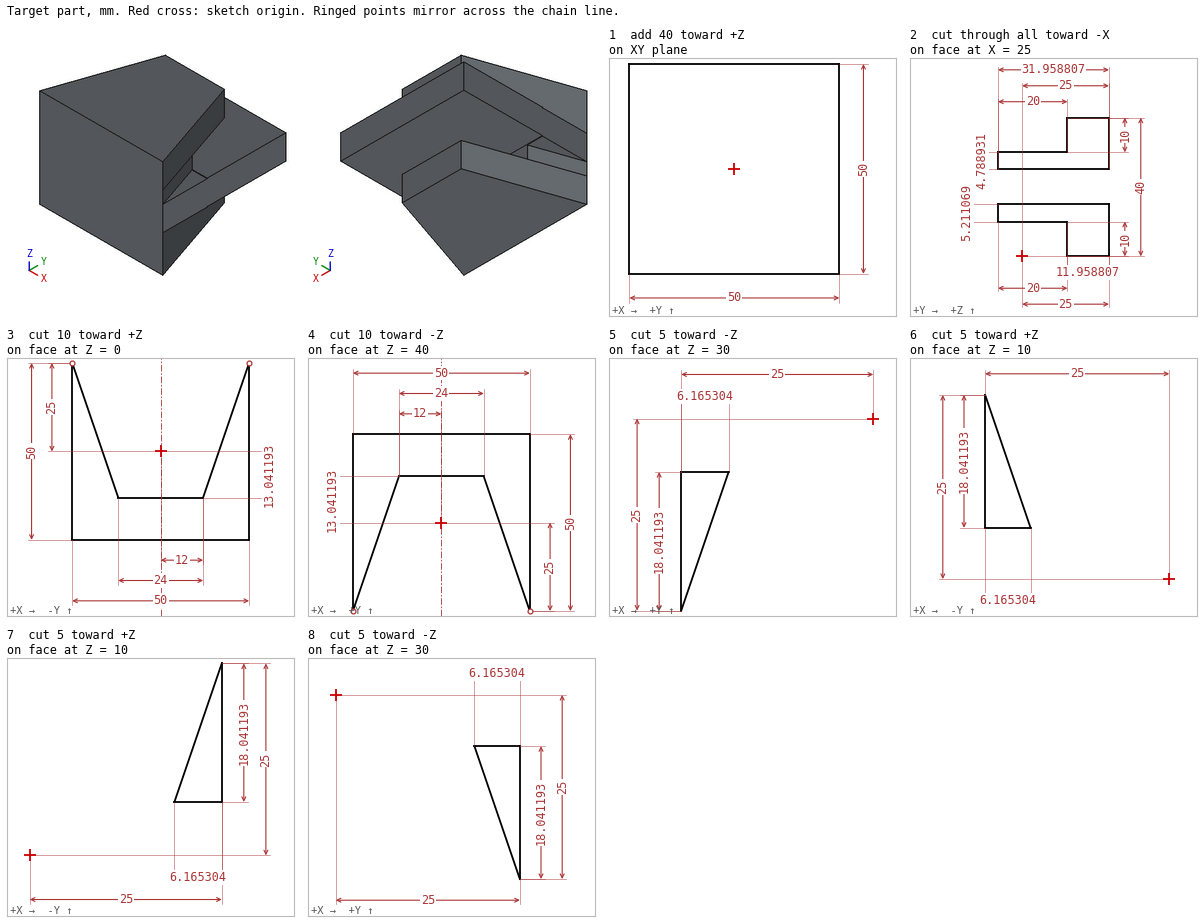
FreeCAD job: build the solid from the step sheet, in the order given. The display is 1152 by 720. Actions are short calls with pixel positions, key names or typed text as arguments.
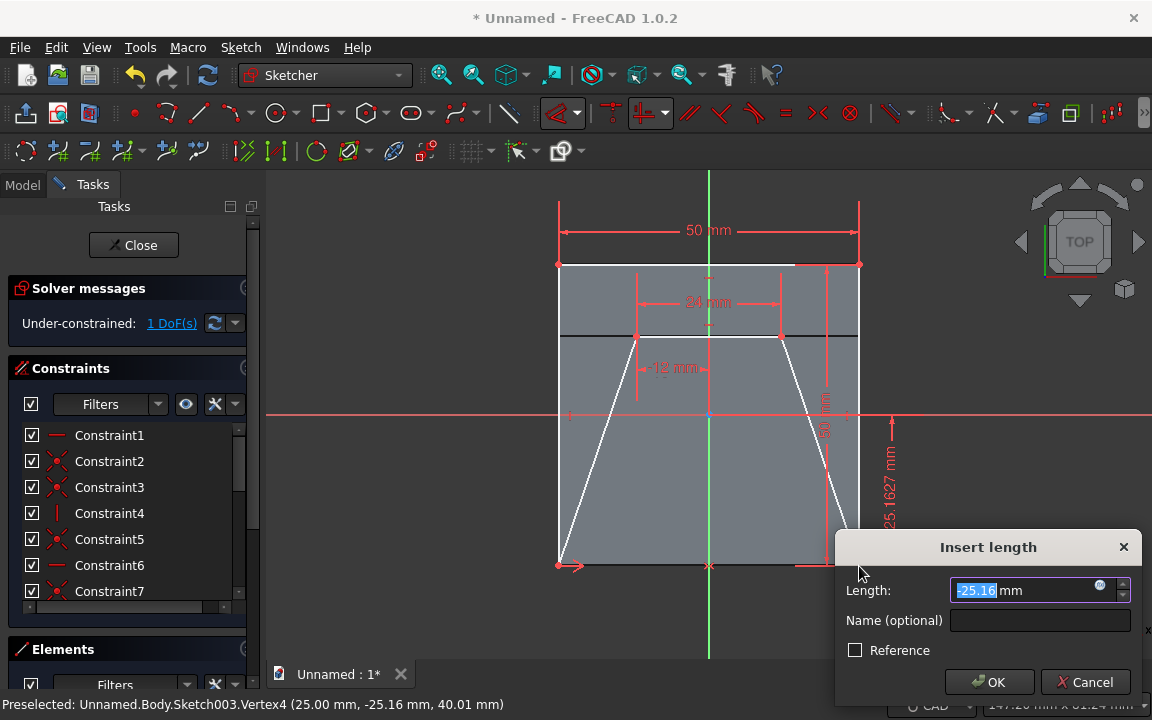
text(-25)
key(Return)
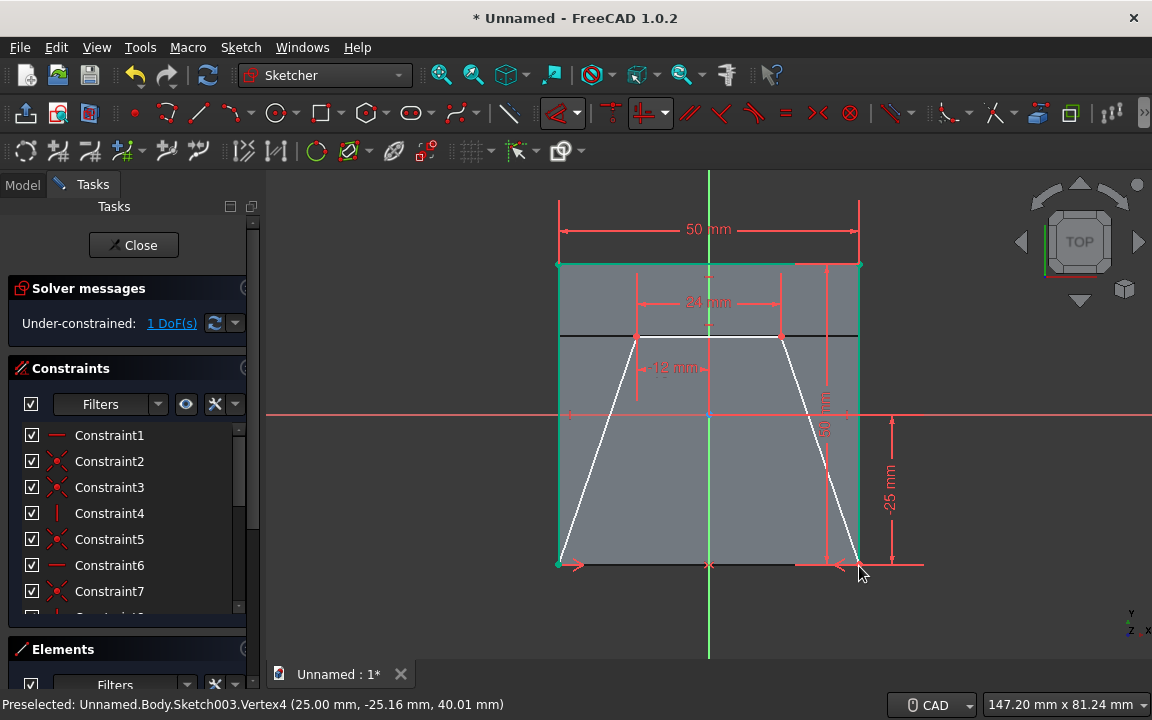
click(637, 337)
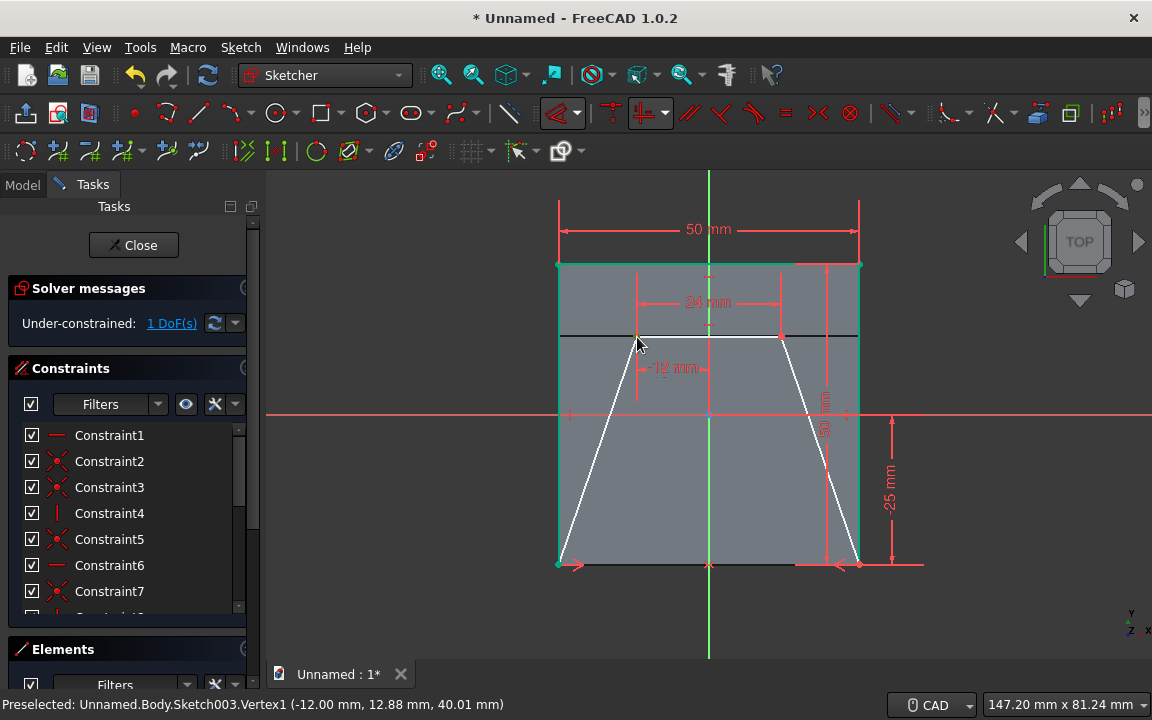
key(i)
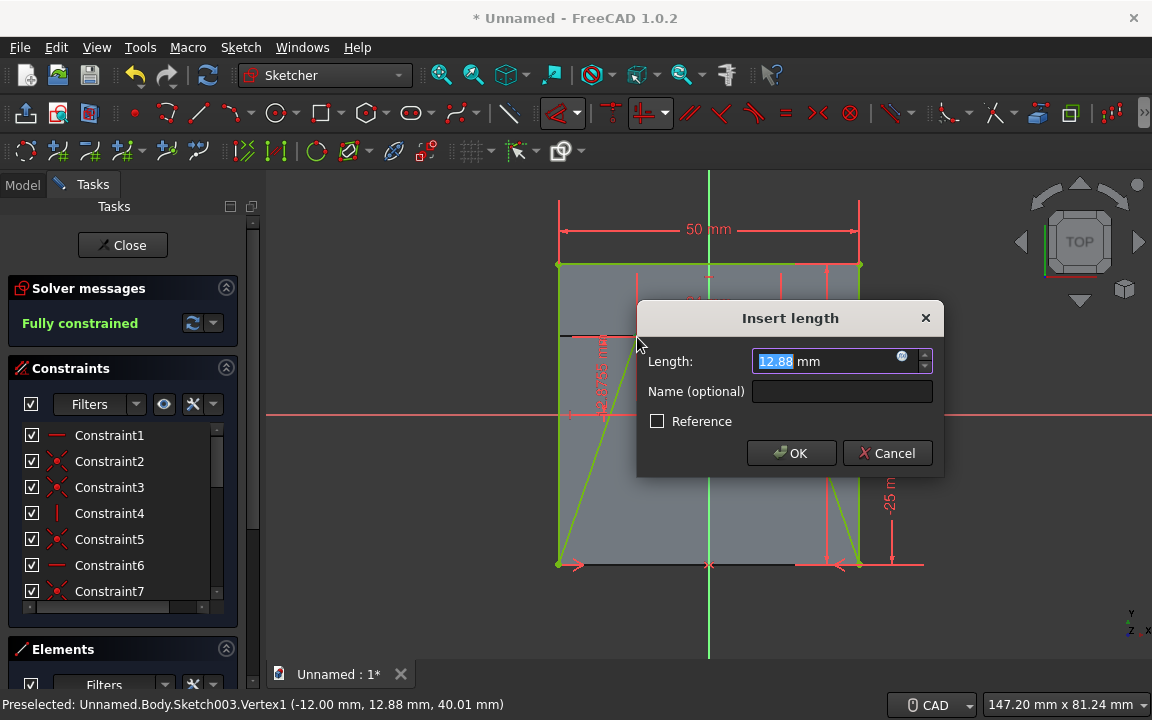
text(13.041193)
key(Return)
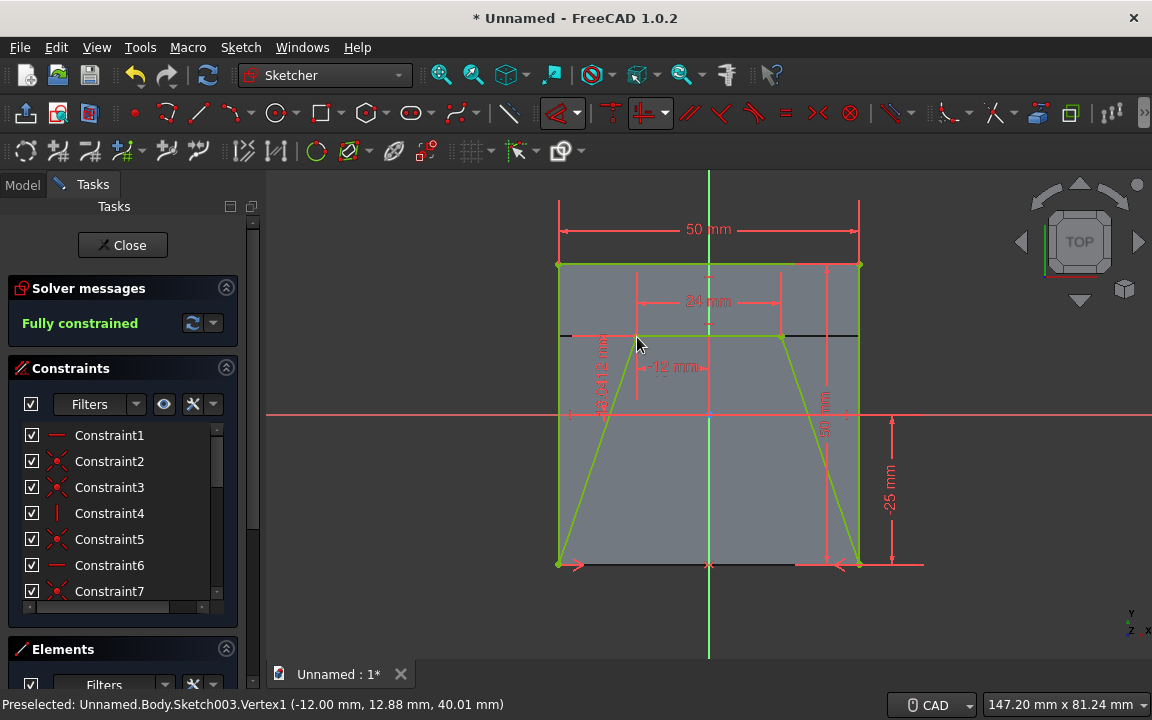
click(123, 245)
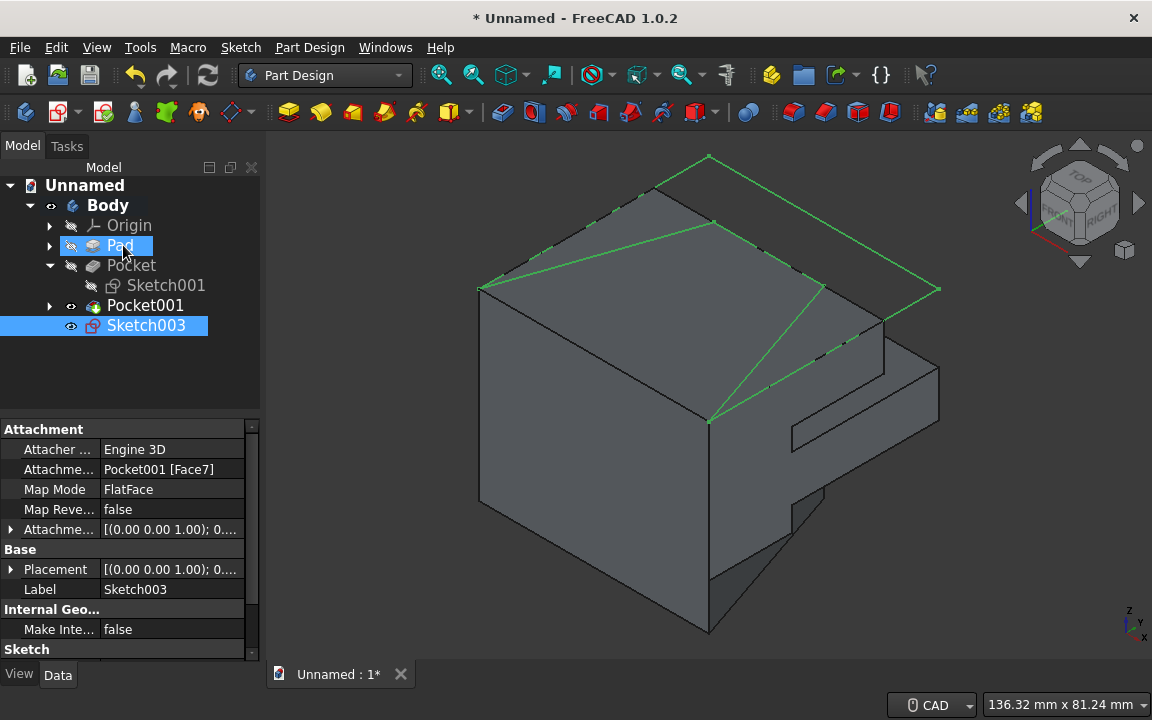
click(504, 112)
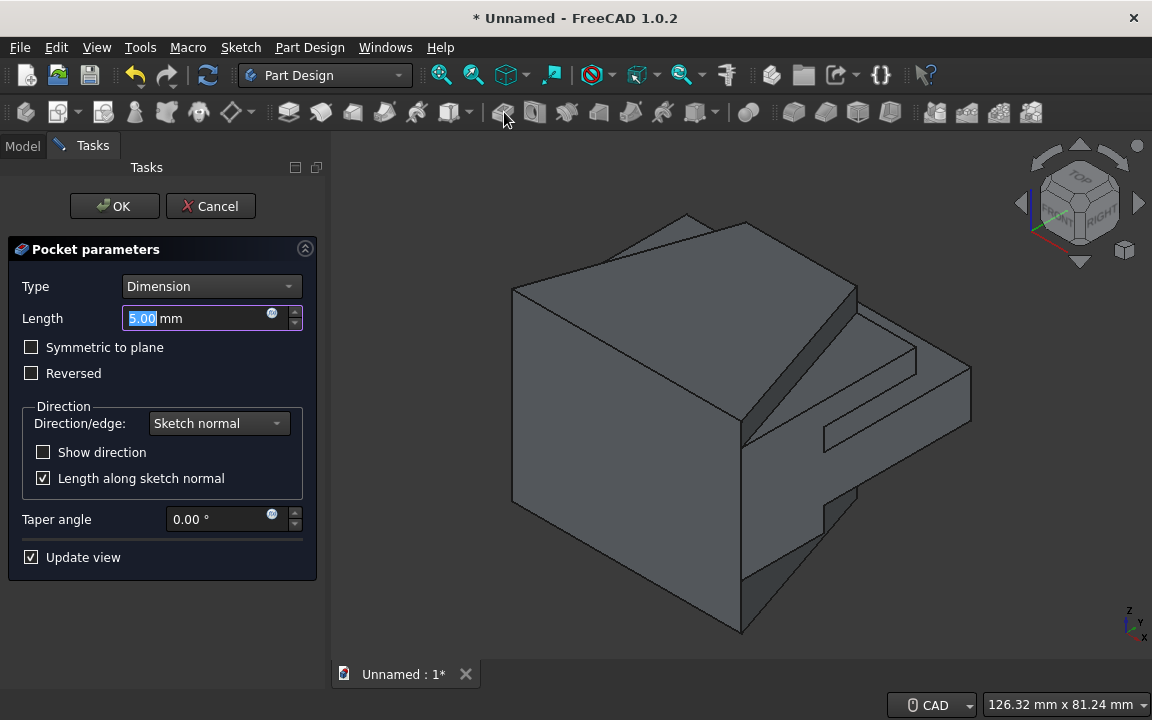
text(10)
key(Tab)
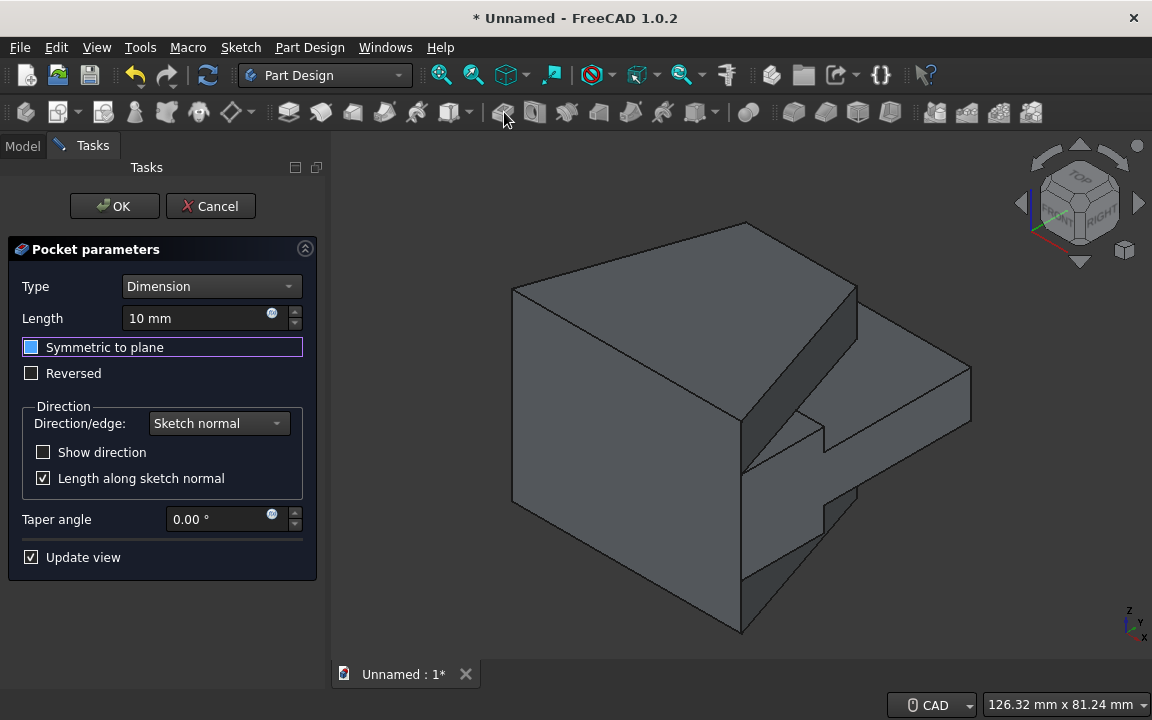
click(115, 206)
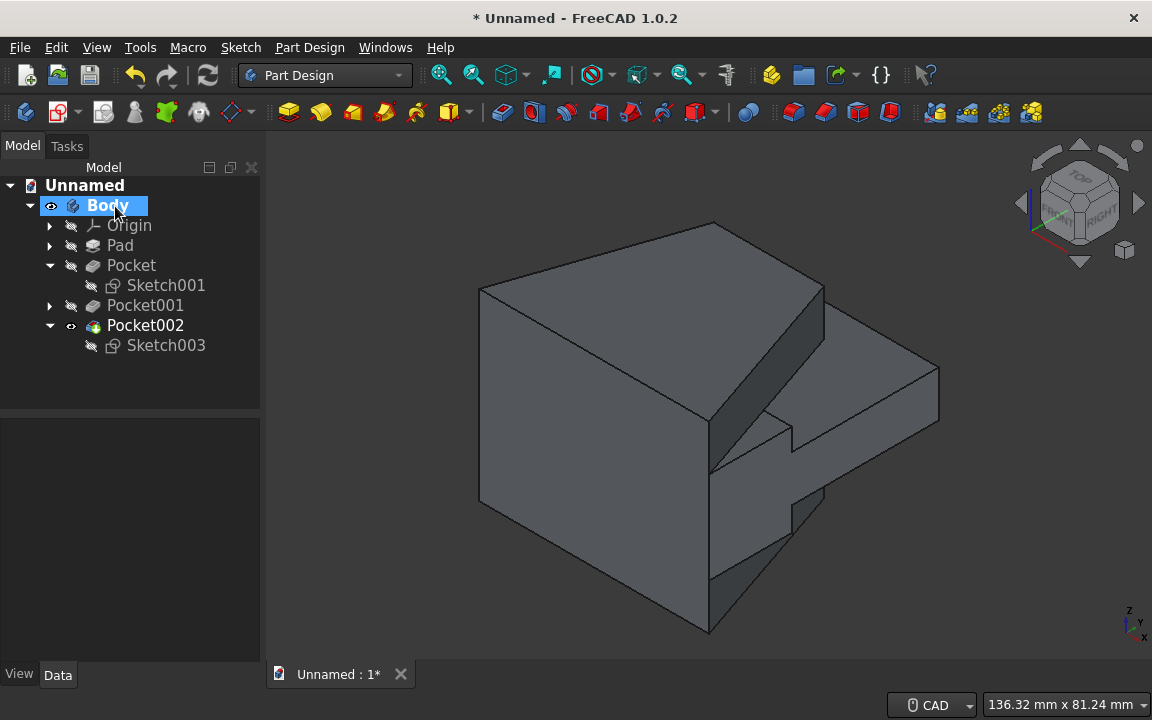
key(2)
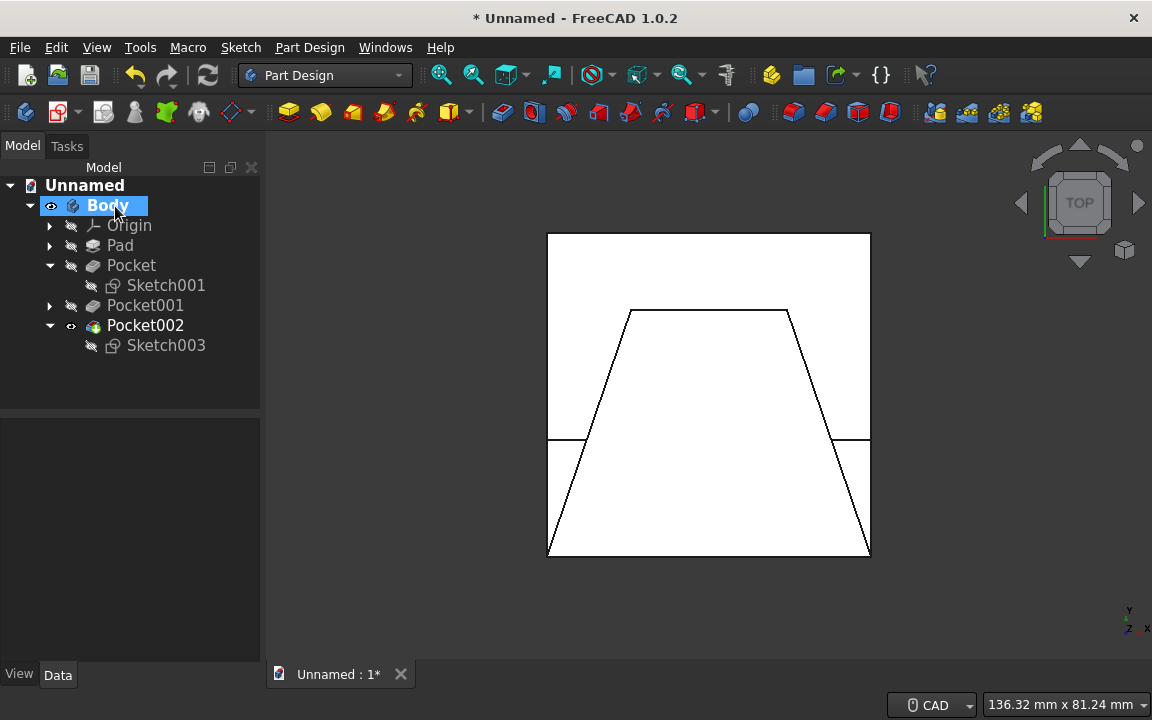
click(561, 464)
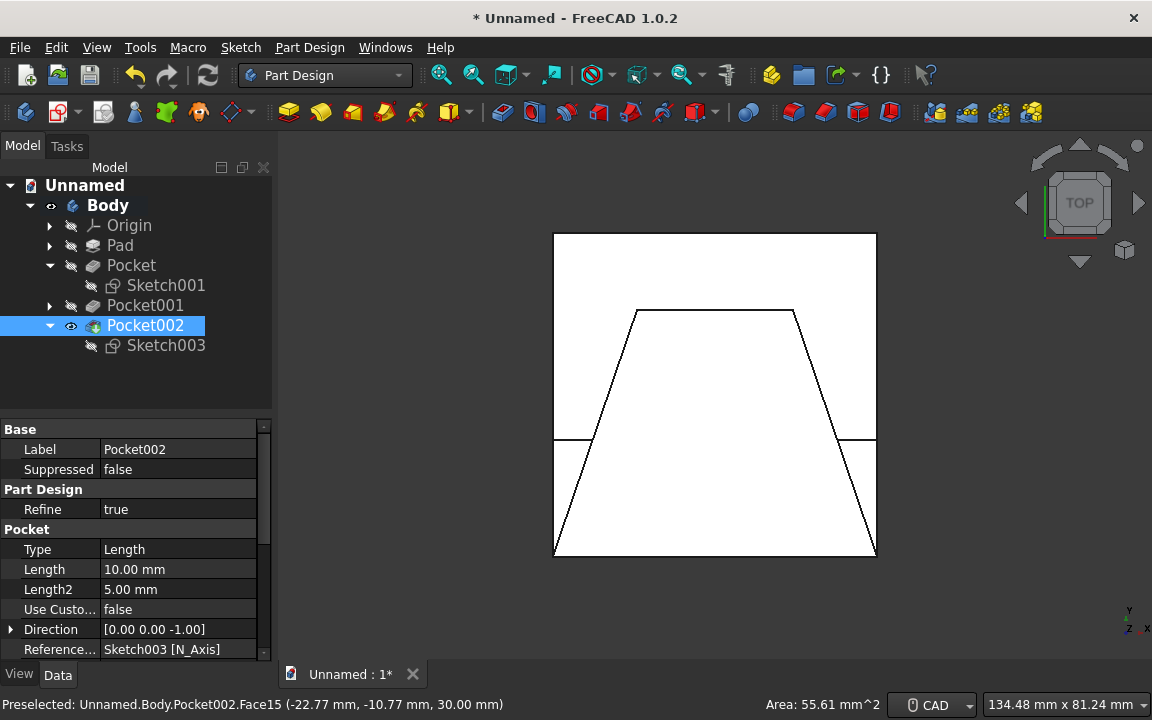
click(58, 112)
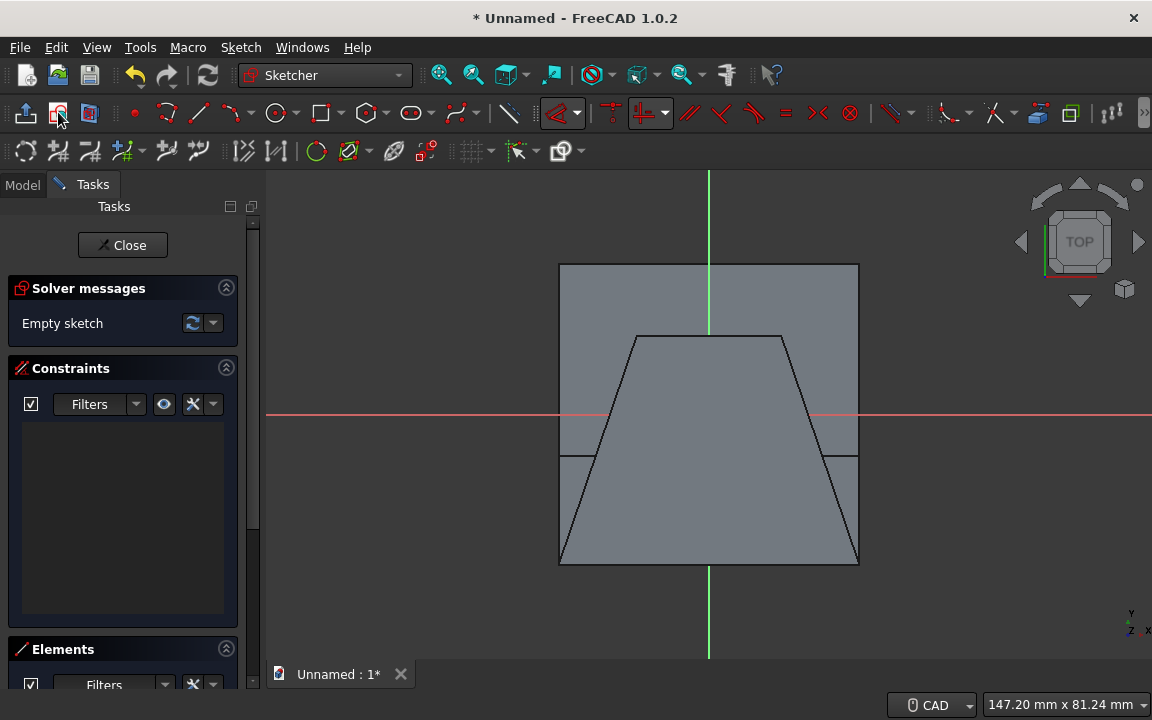
click(90, 114)